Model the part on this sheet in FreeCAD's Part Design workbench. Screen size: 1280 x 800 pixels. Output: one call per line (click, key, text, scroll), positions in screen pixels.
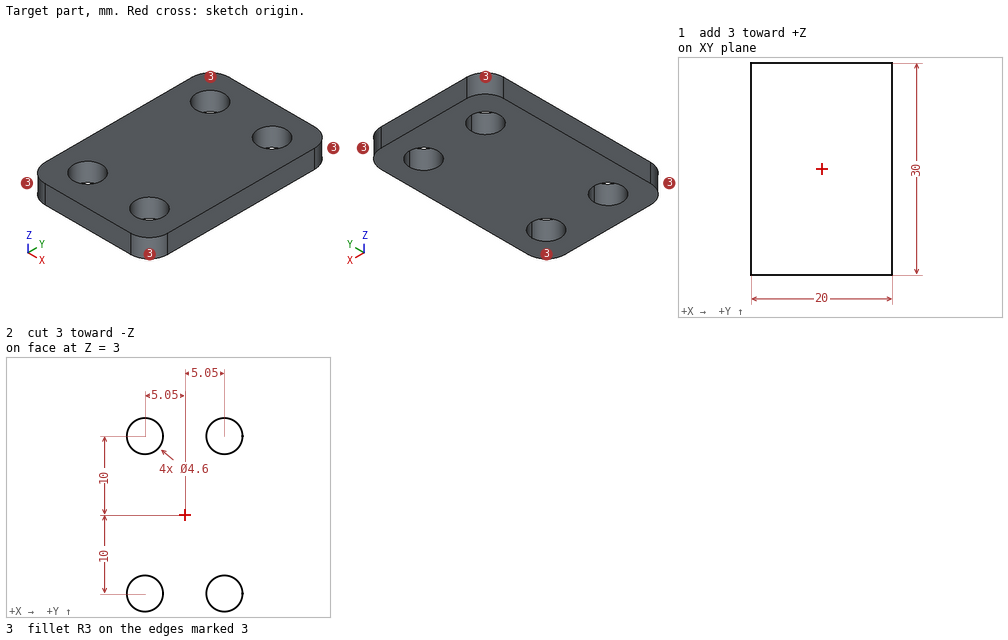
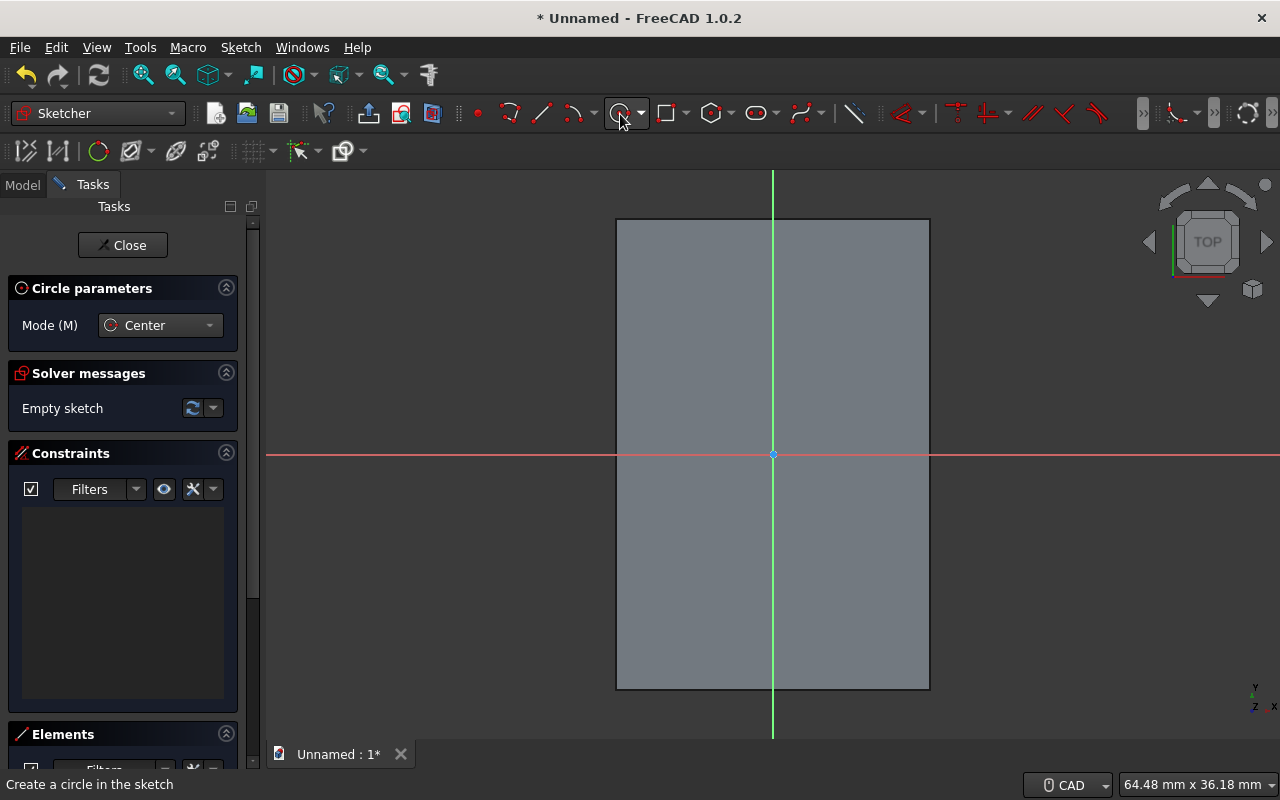
click(694, 297)
click(719, 272)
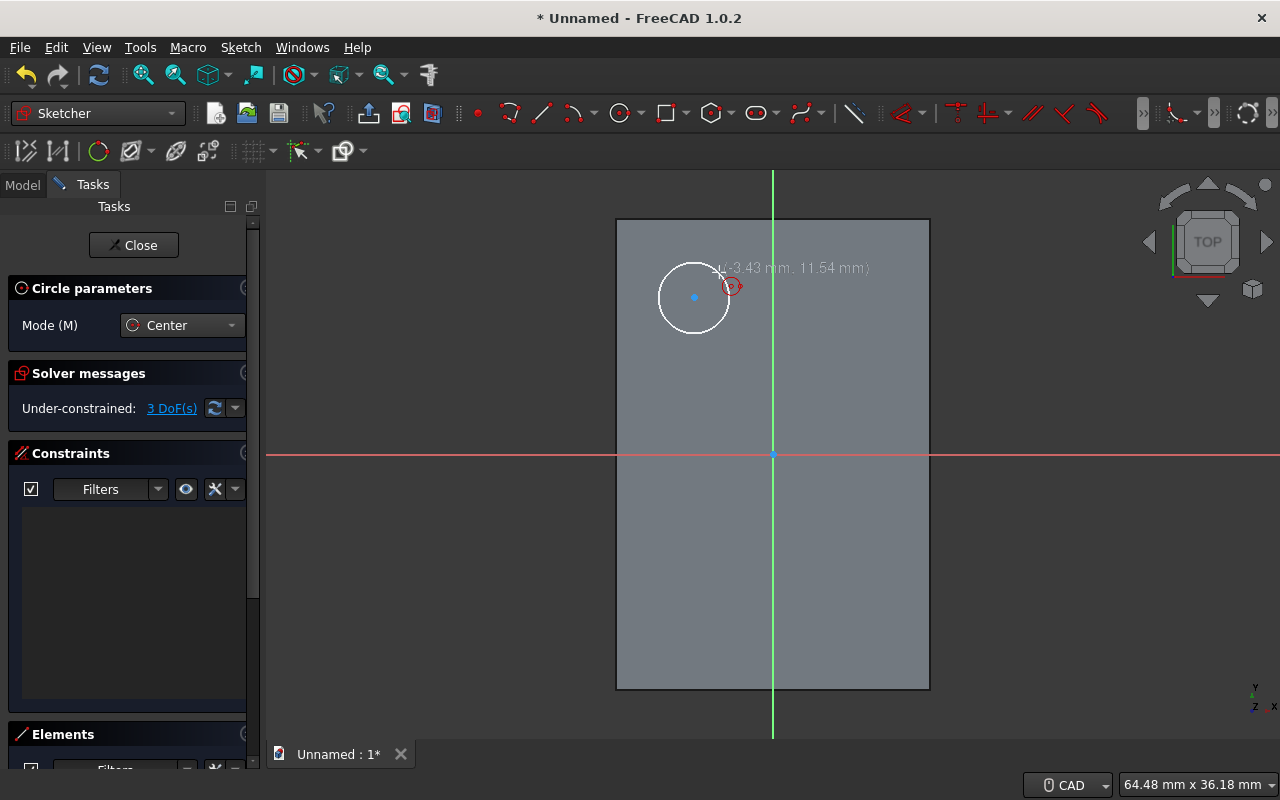
click(852, 297)
click(878, 272)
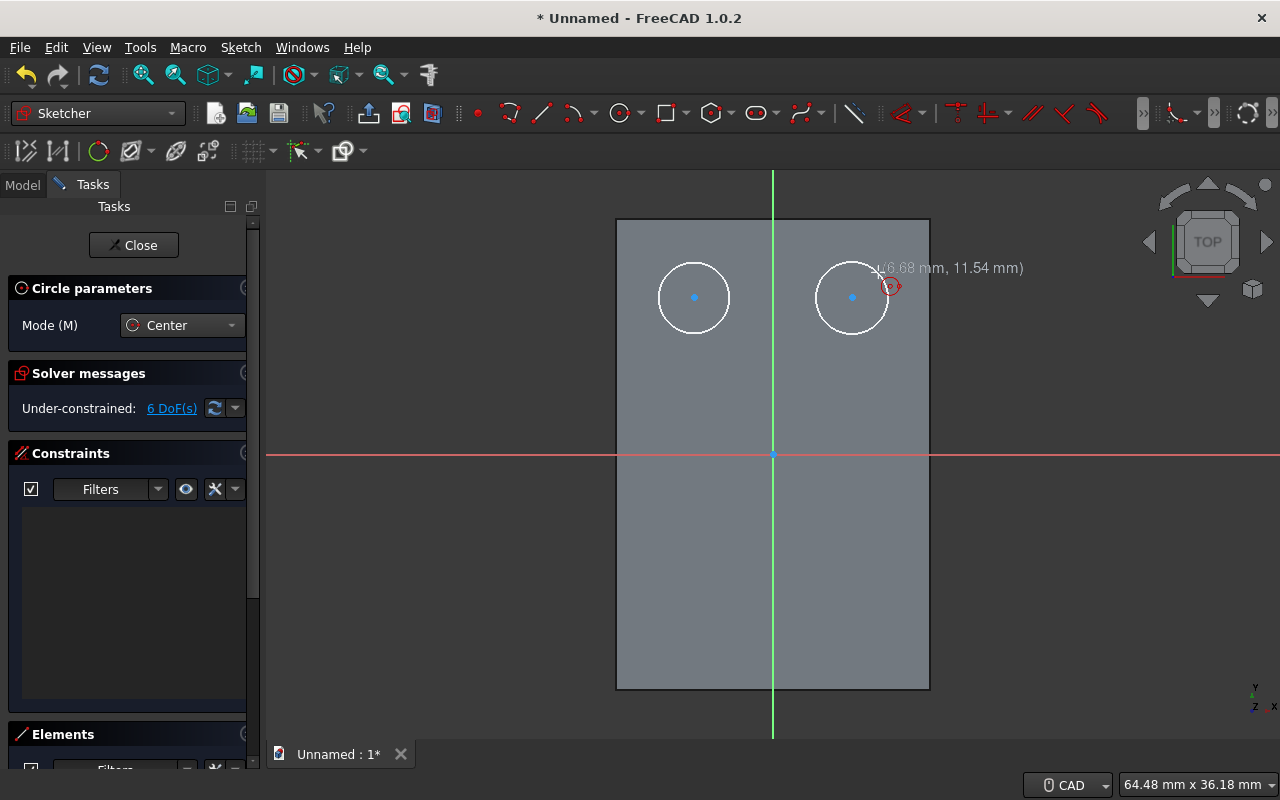
click(694, 612)
click(719, 586)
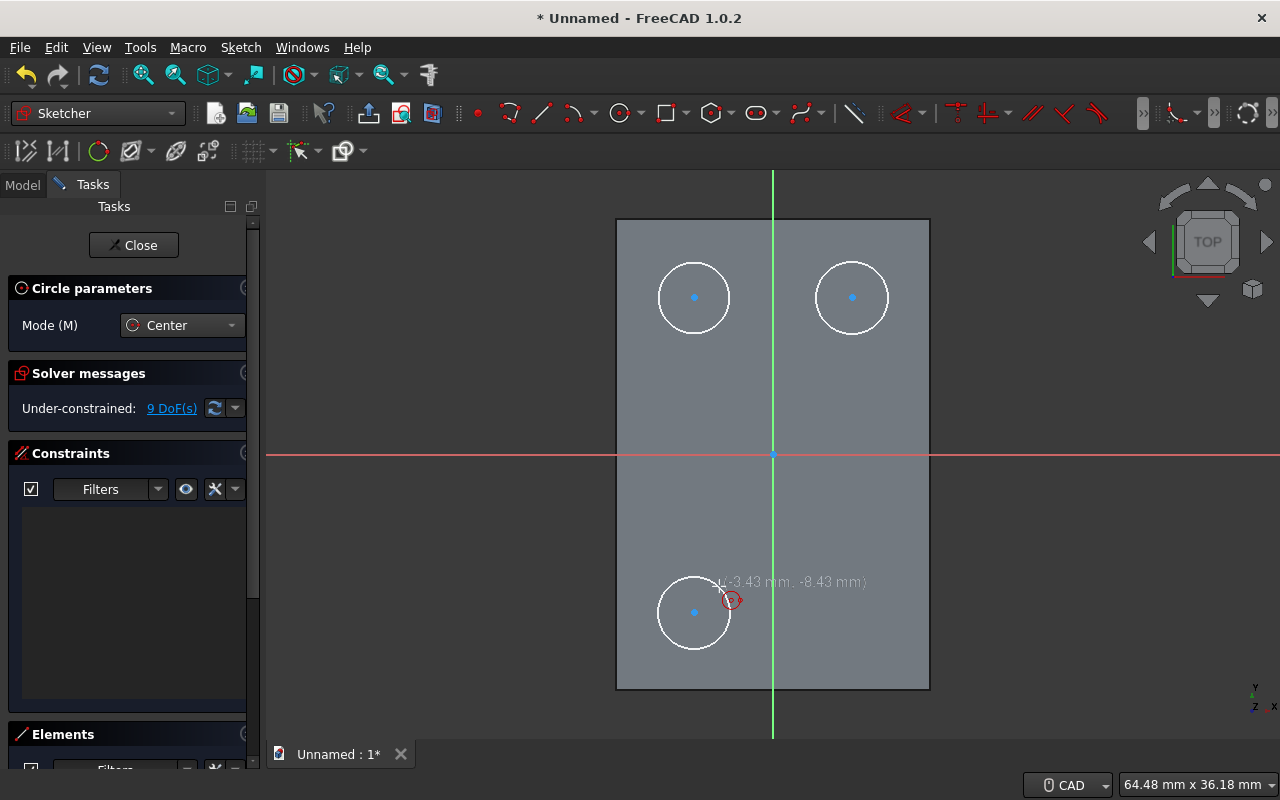
click(852, 612)
click(878, 586)
key(Escape)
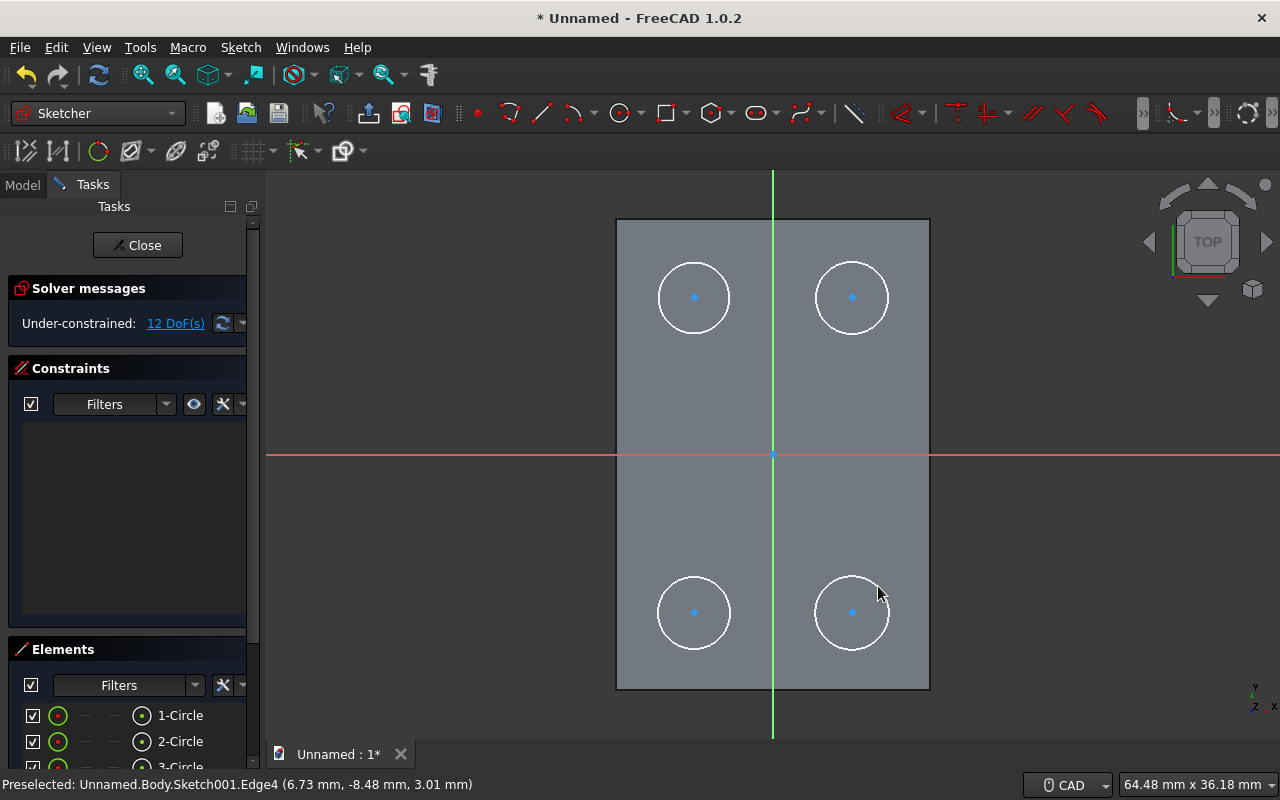
click(719, 273)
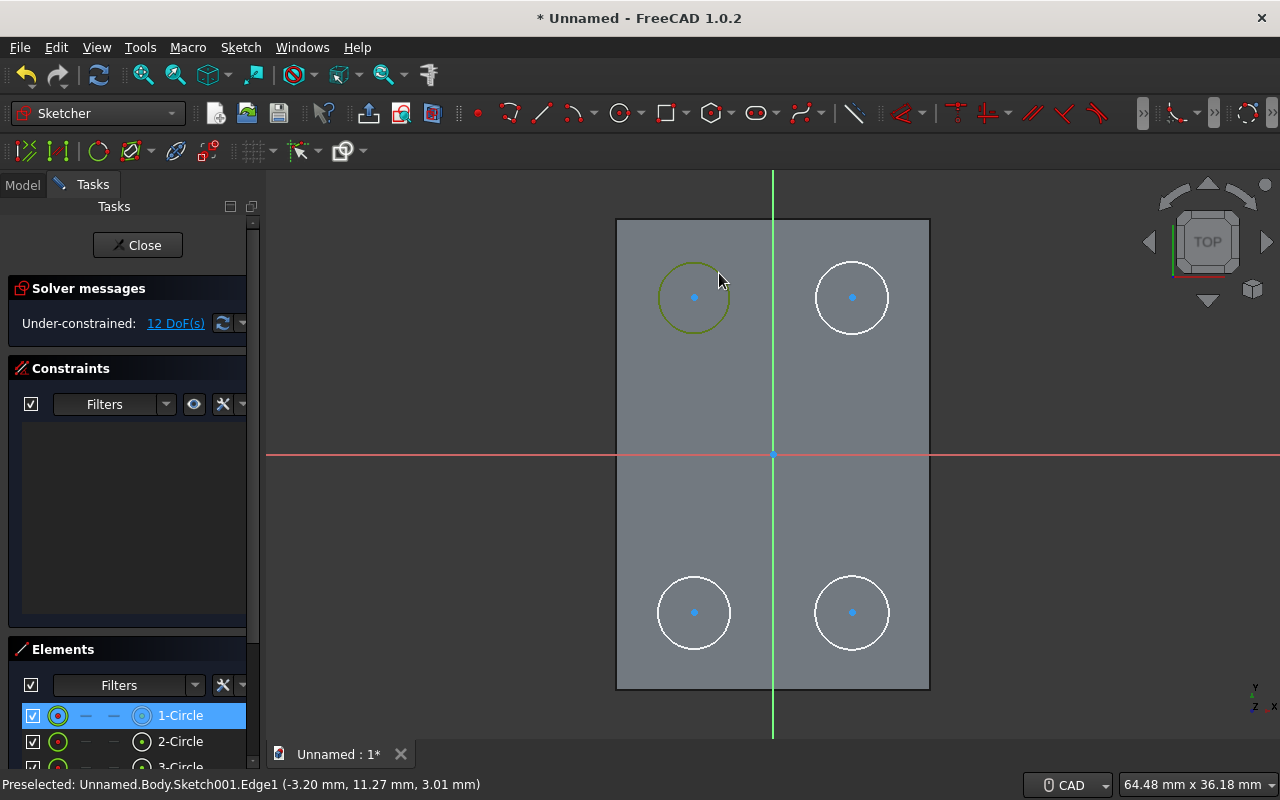
click(877, 272)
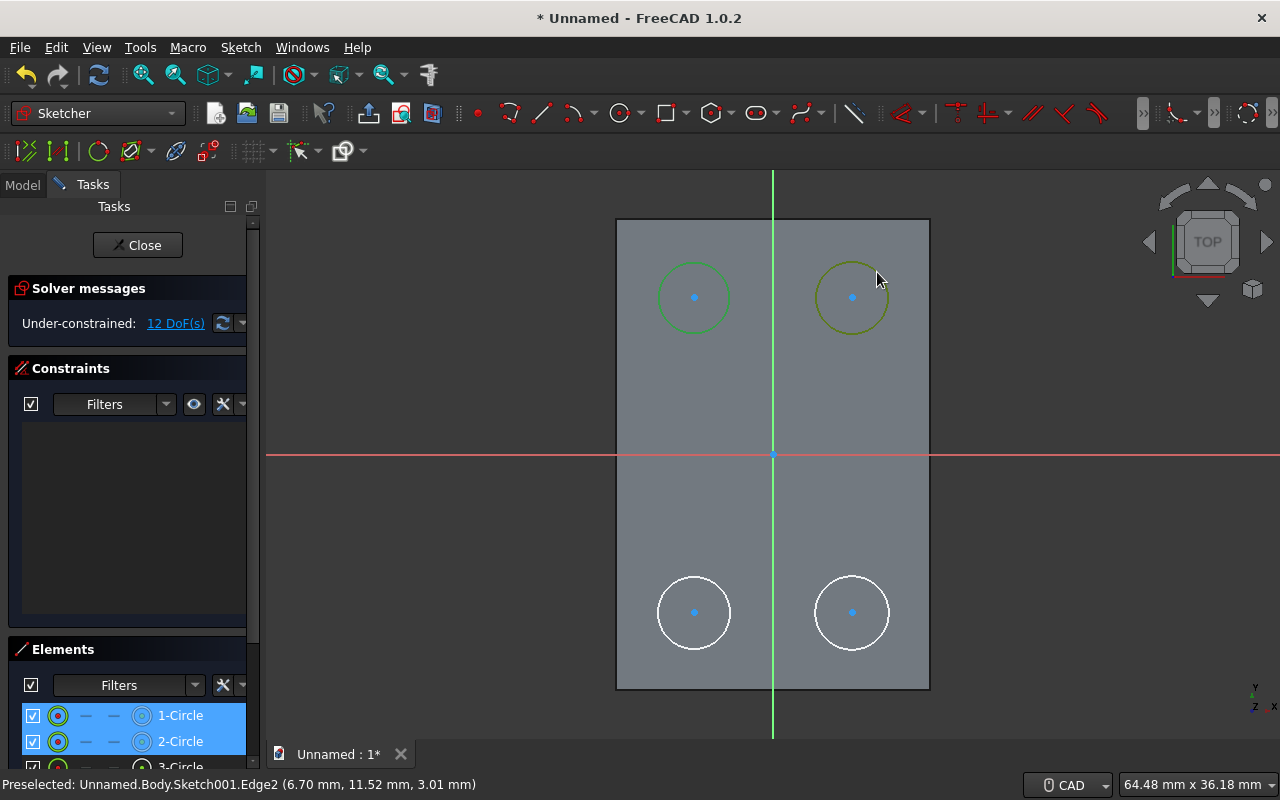
click(719, 587)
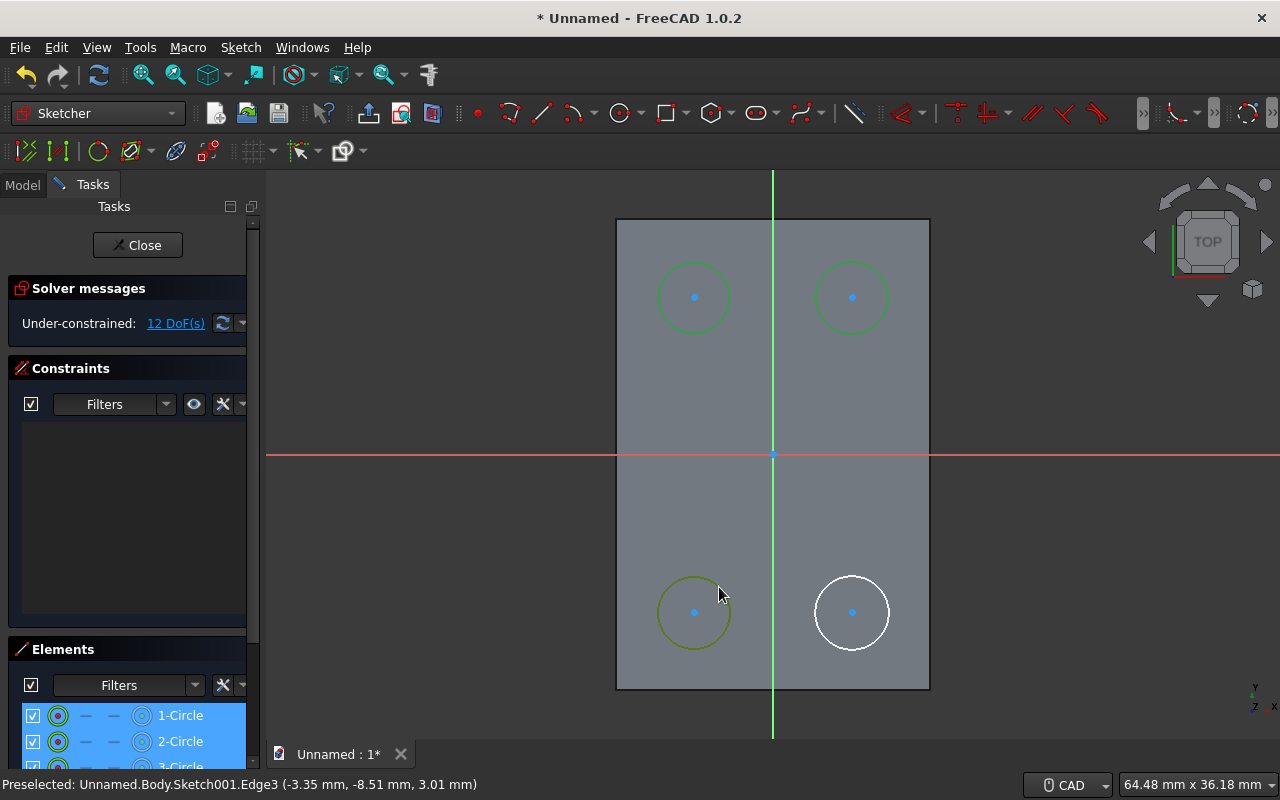
click(878, 587)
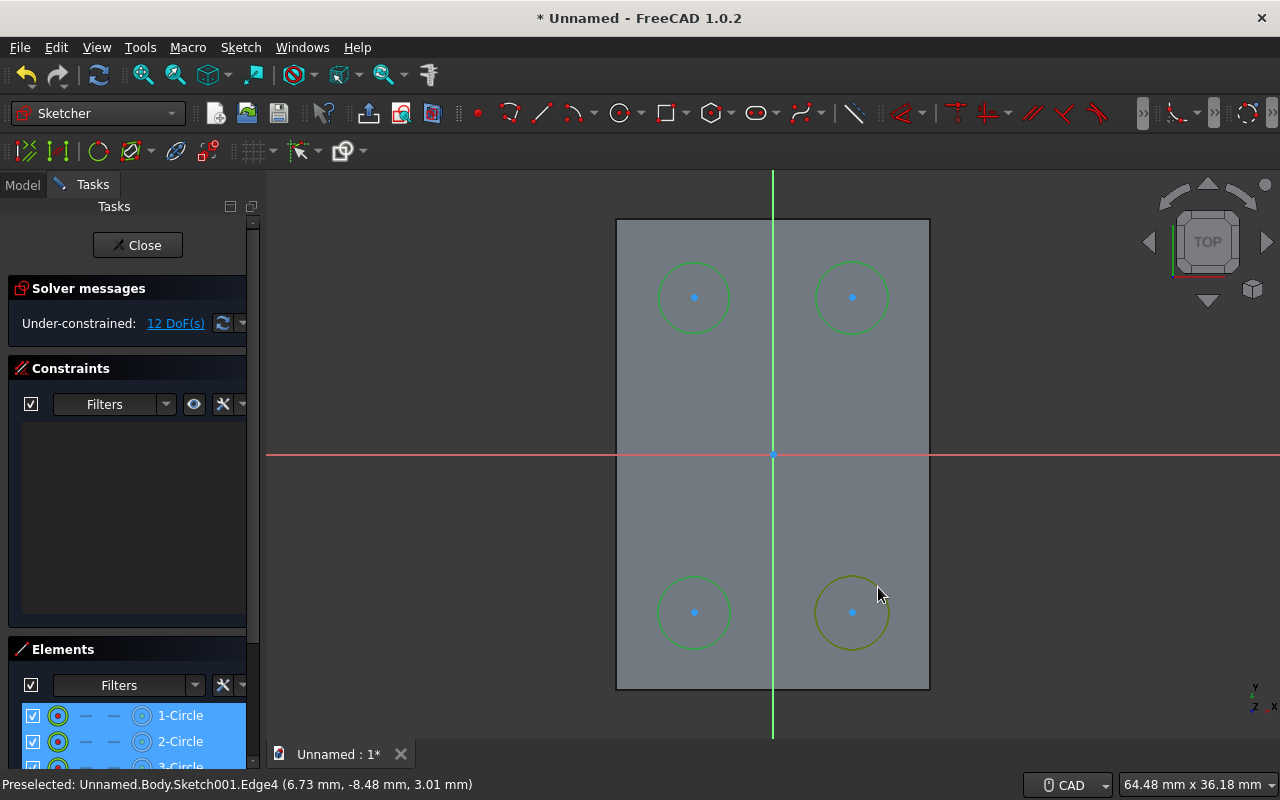
key(e)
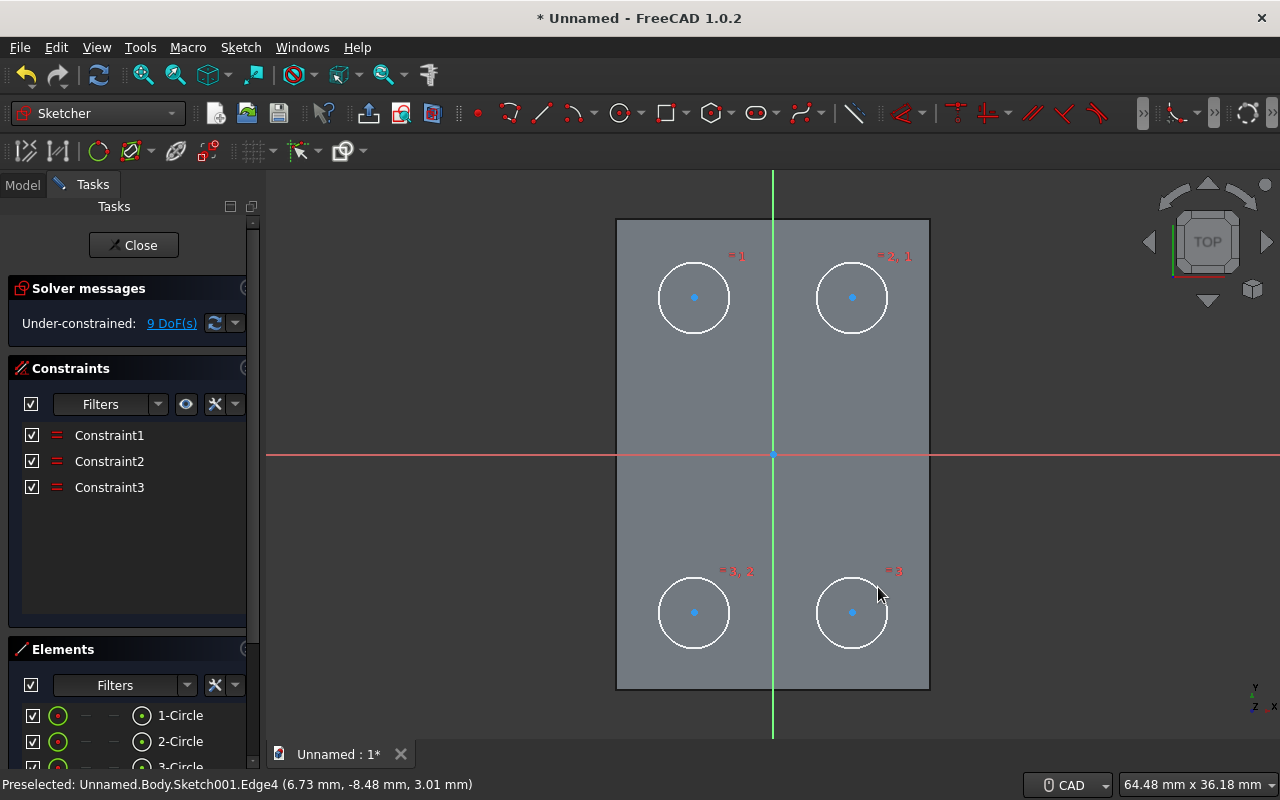
click(694, 298)